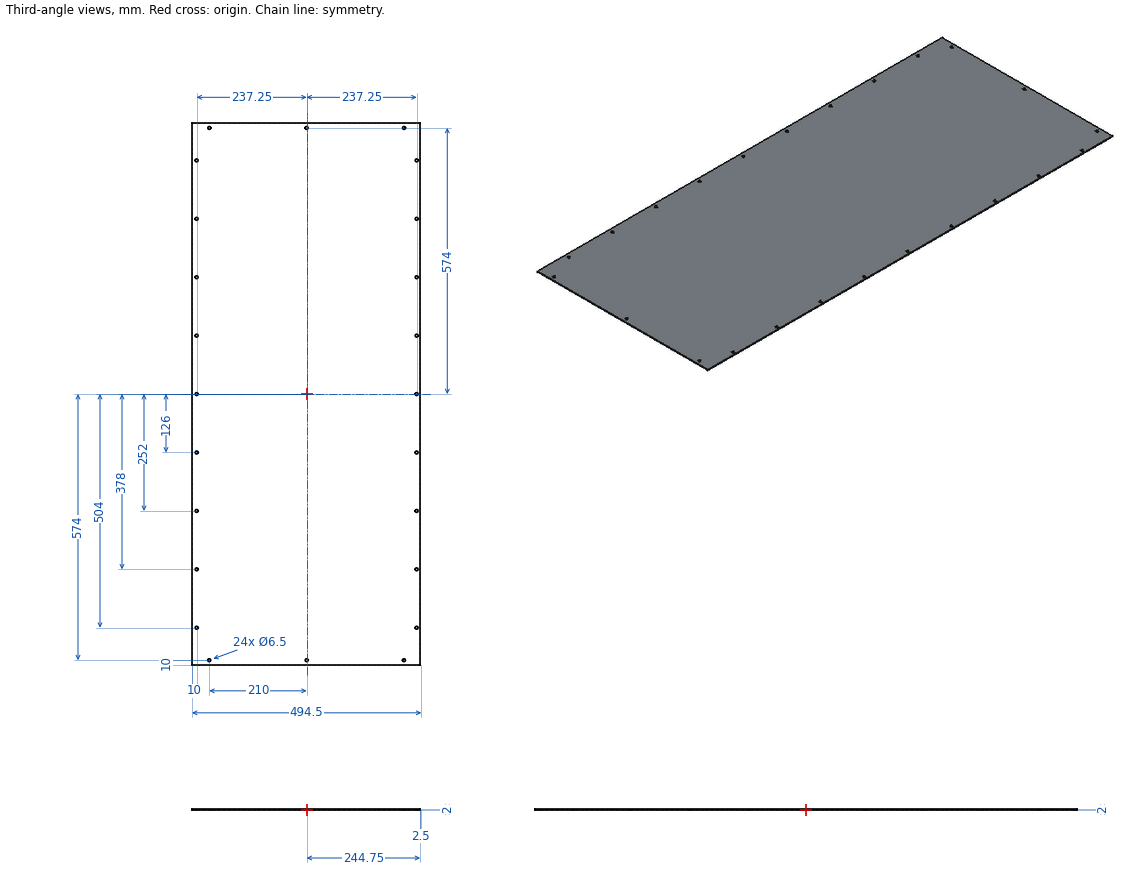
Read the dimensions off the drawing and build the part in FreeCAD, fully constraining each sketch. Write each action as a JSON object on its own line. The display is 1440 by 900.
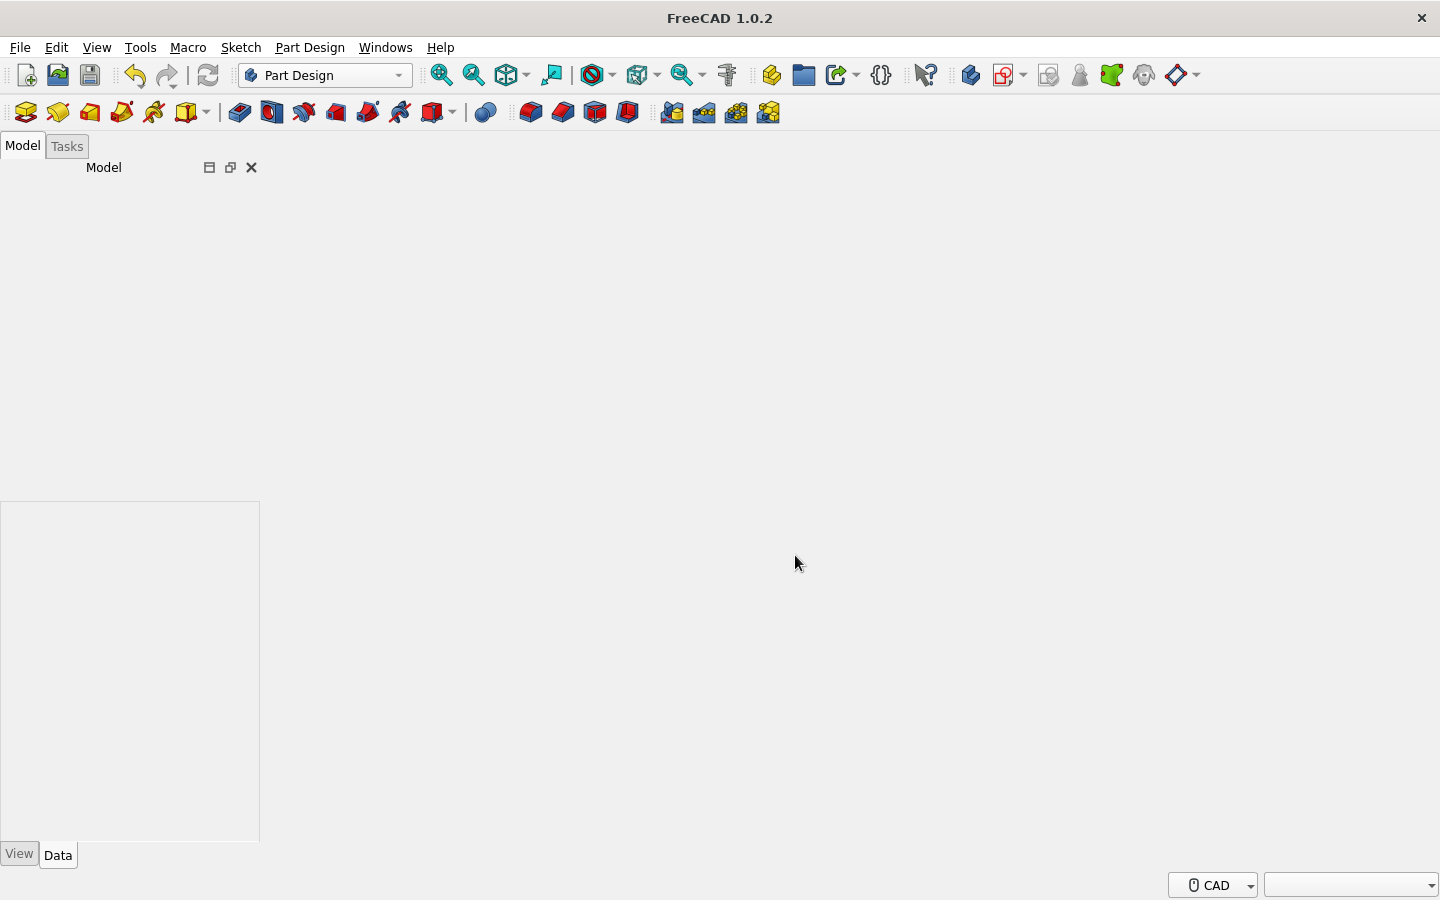
{"action": "key", "text": "ctrl+n"}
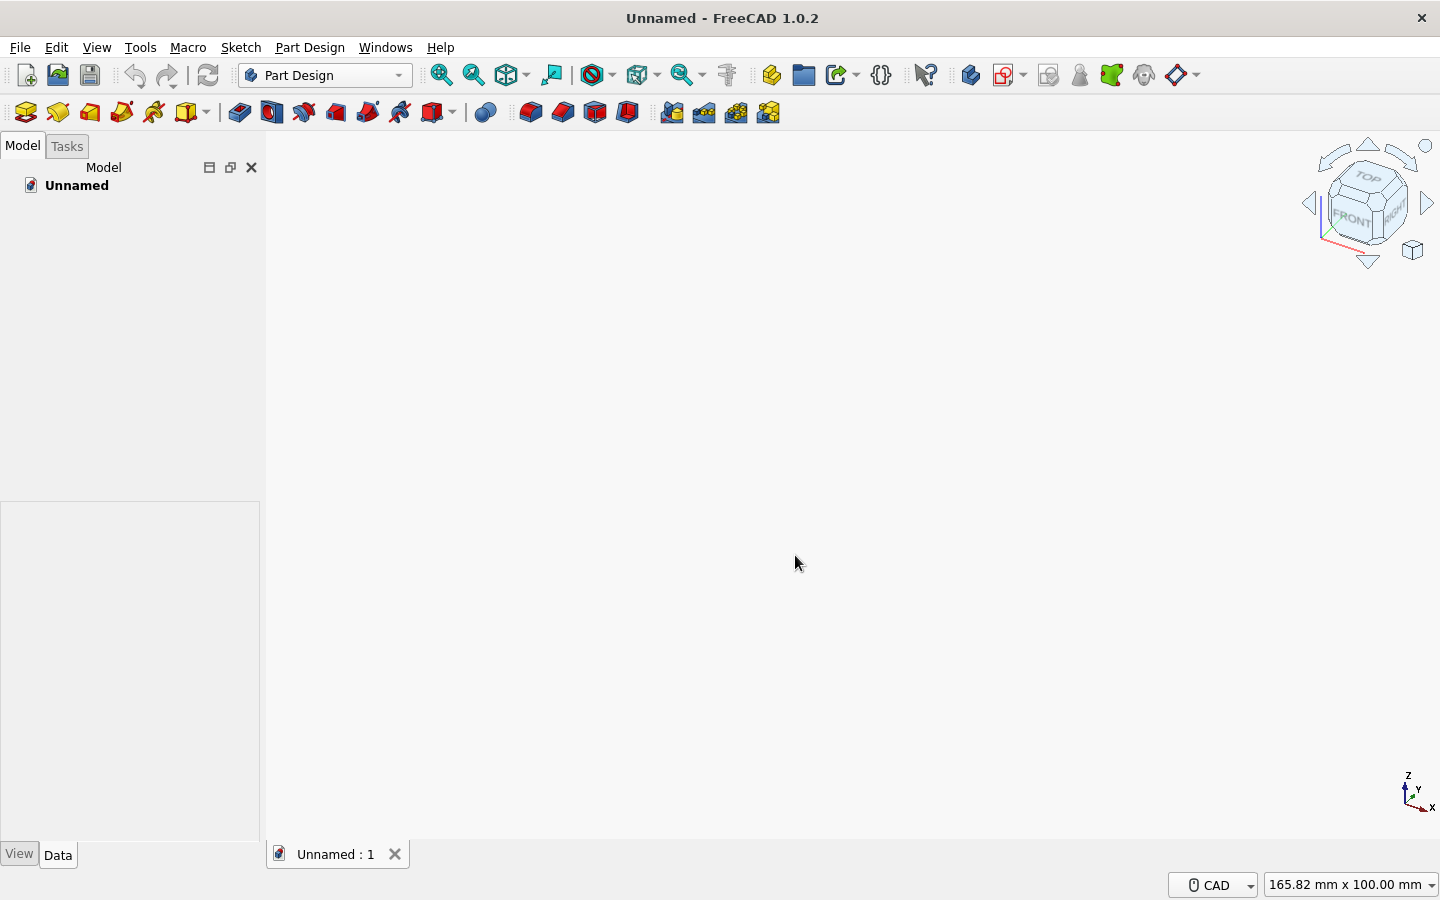
{"action": "left_click", "coordinate": [1004, 76]}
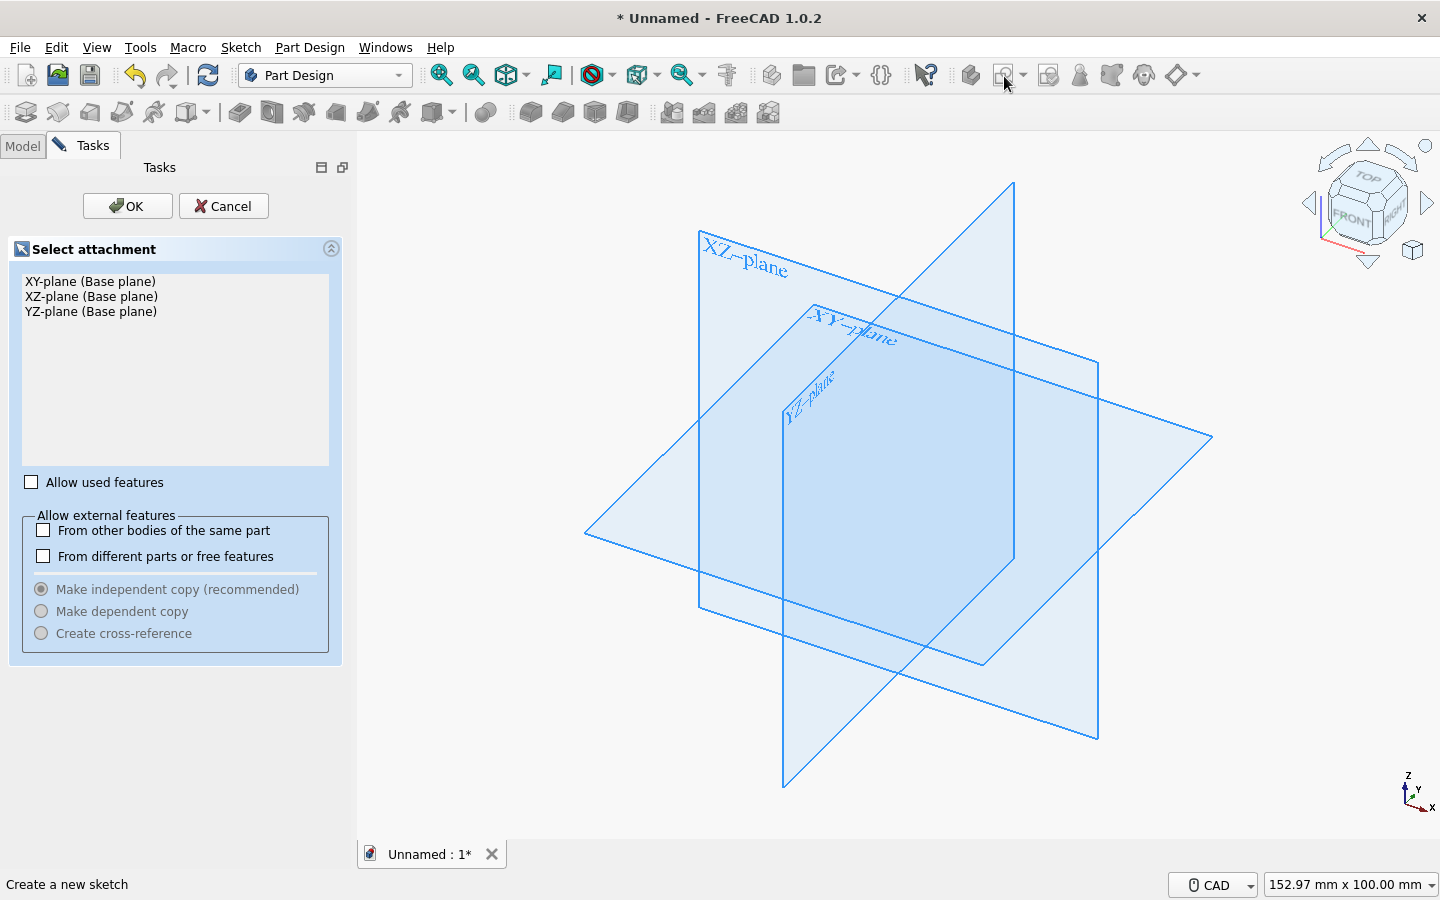
{"action": "left_click", "coordinate": [82, 282]}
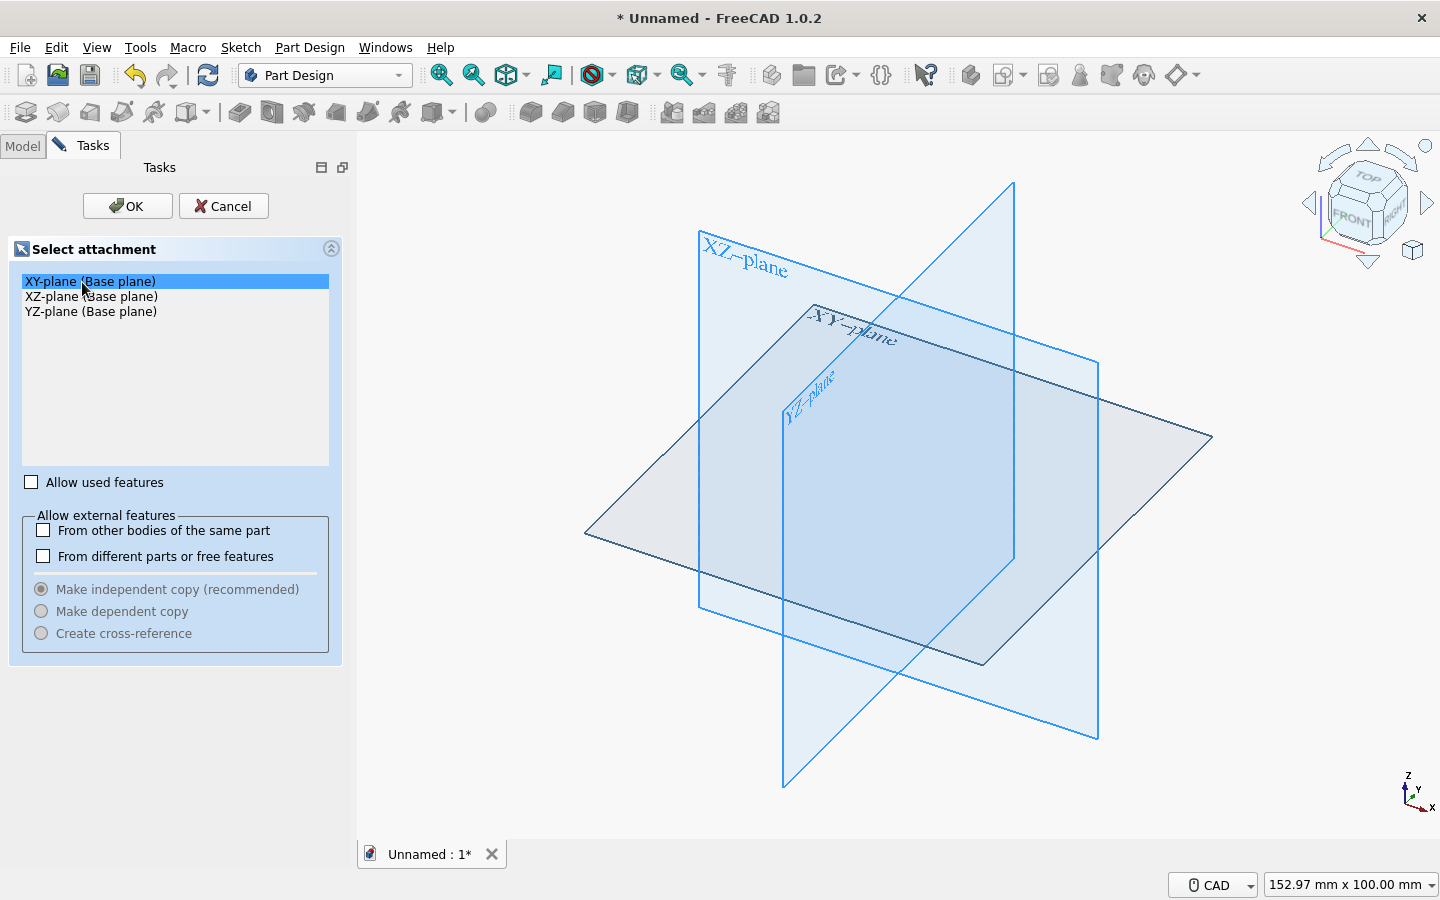
{"action": "left_click", "coordinate": [128, 206]}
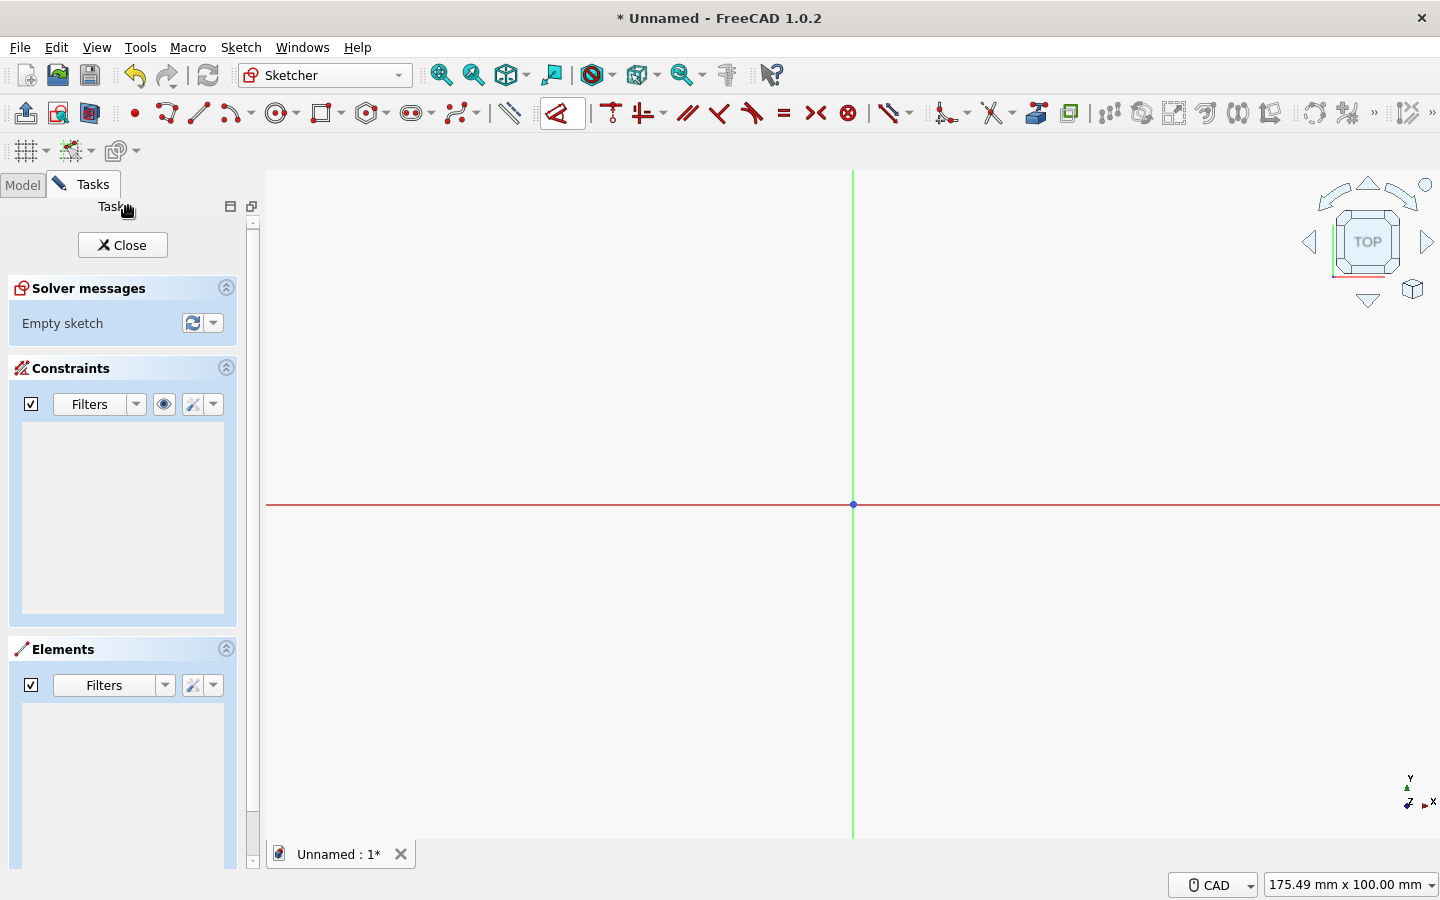
{"action": "scroll", "coordinate": [780, 504], "scroll_direction": "down", "scroll_amount": 14}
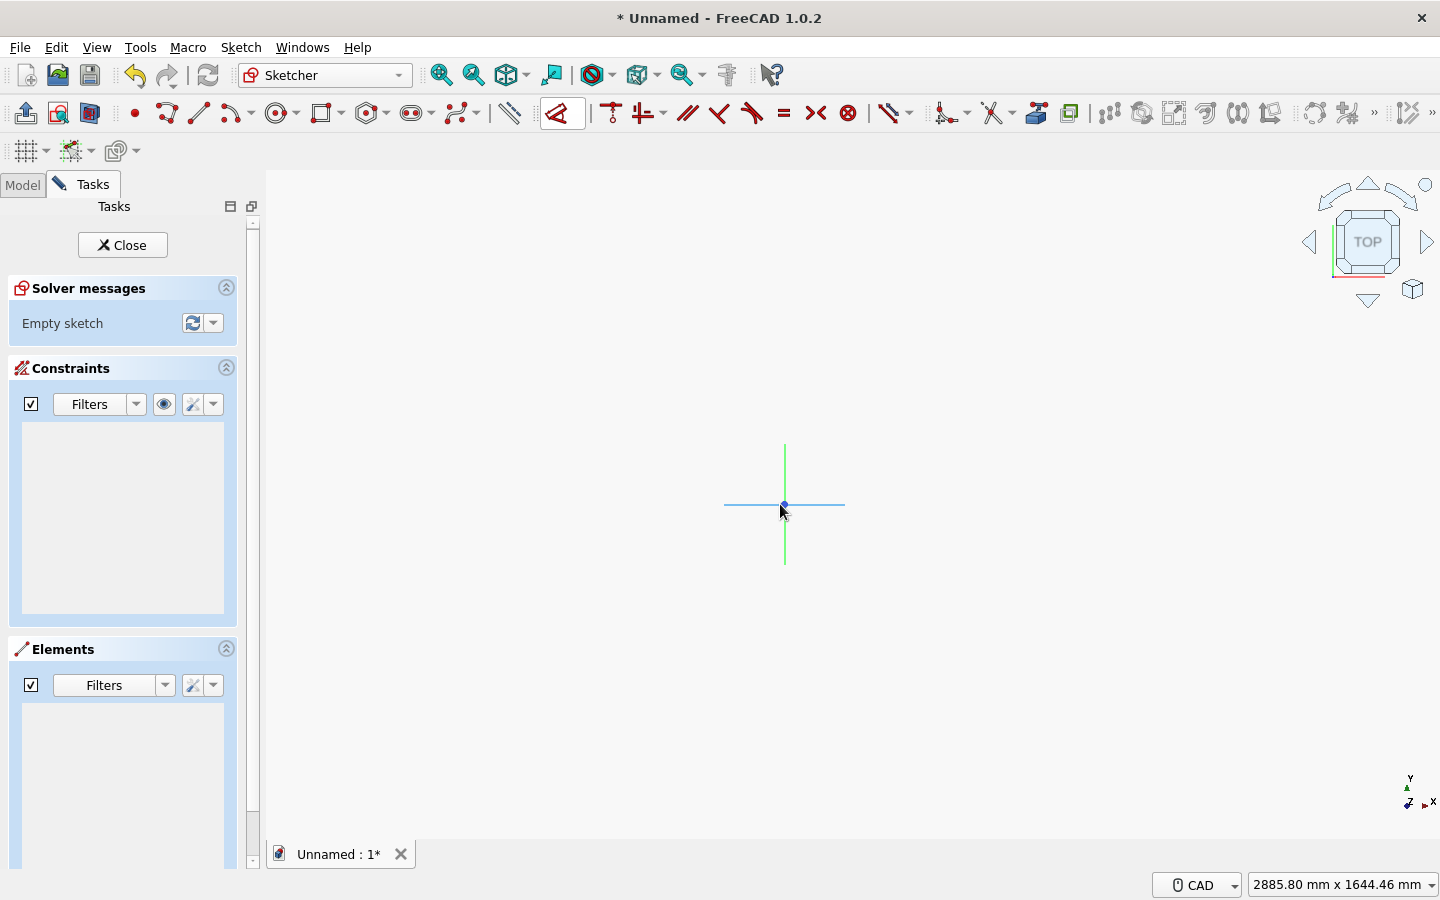
{"action": "key", "text": "g v"}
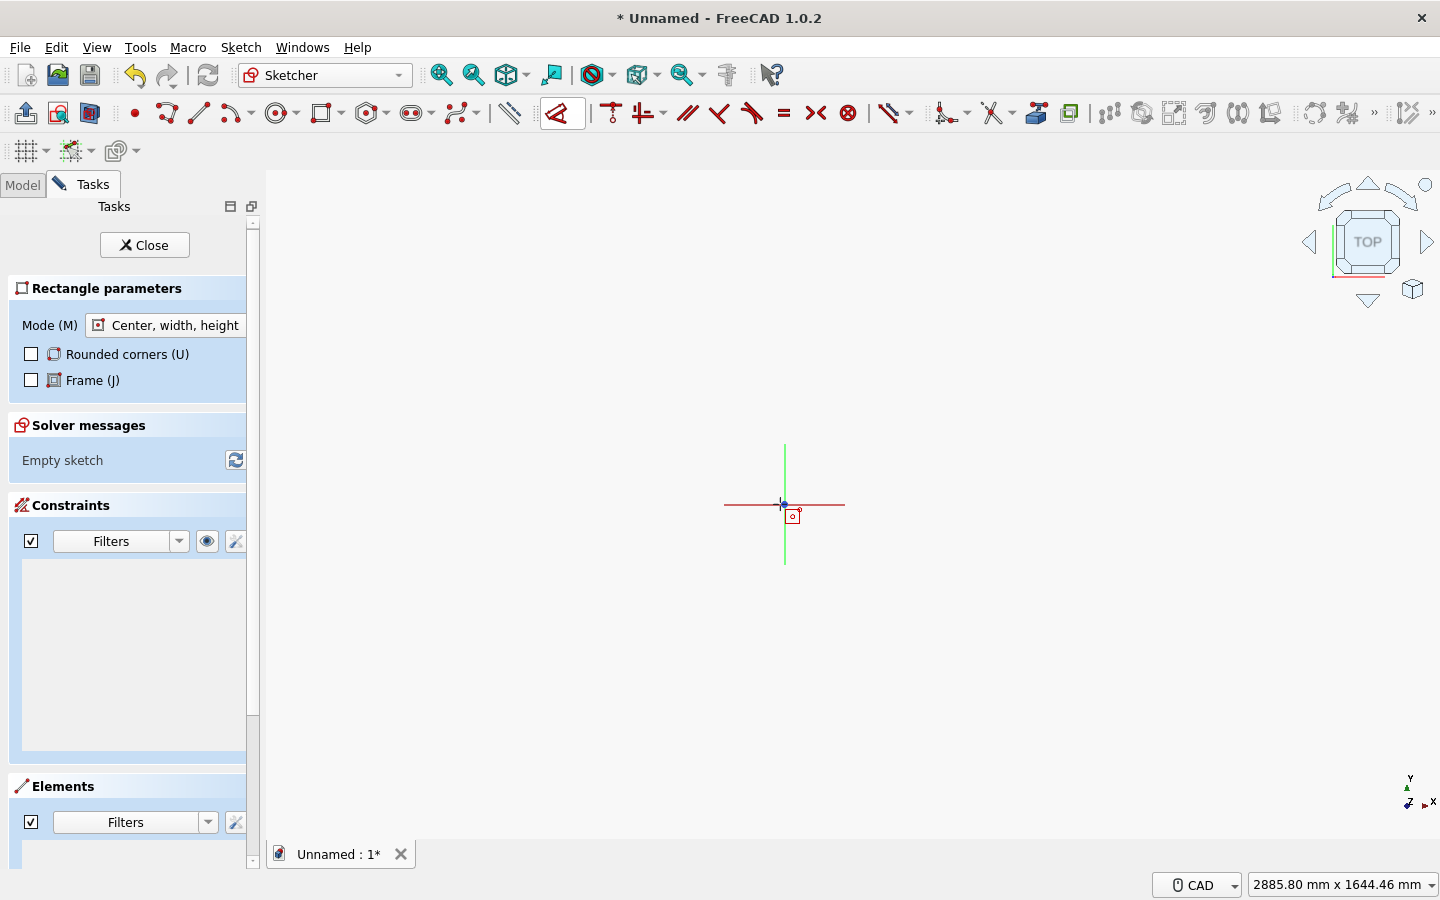
{"action": "left_click", "coordinate": [785, 504]}
{"action": "left_click", "coordinate": [885, 267]}